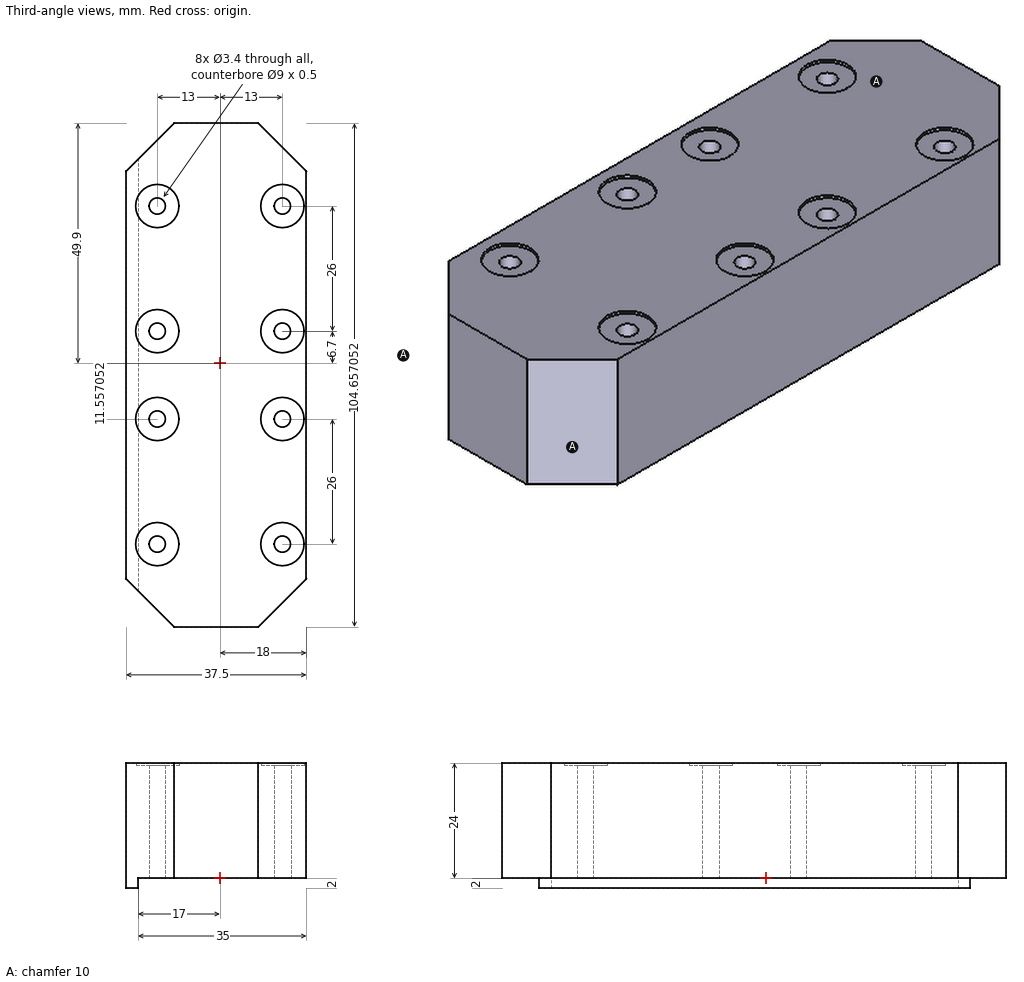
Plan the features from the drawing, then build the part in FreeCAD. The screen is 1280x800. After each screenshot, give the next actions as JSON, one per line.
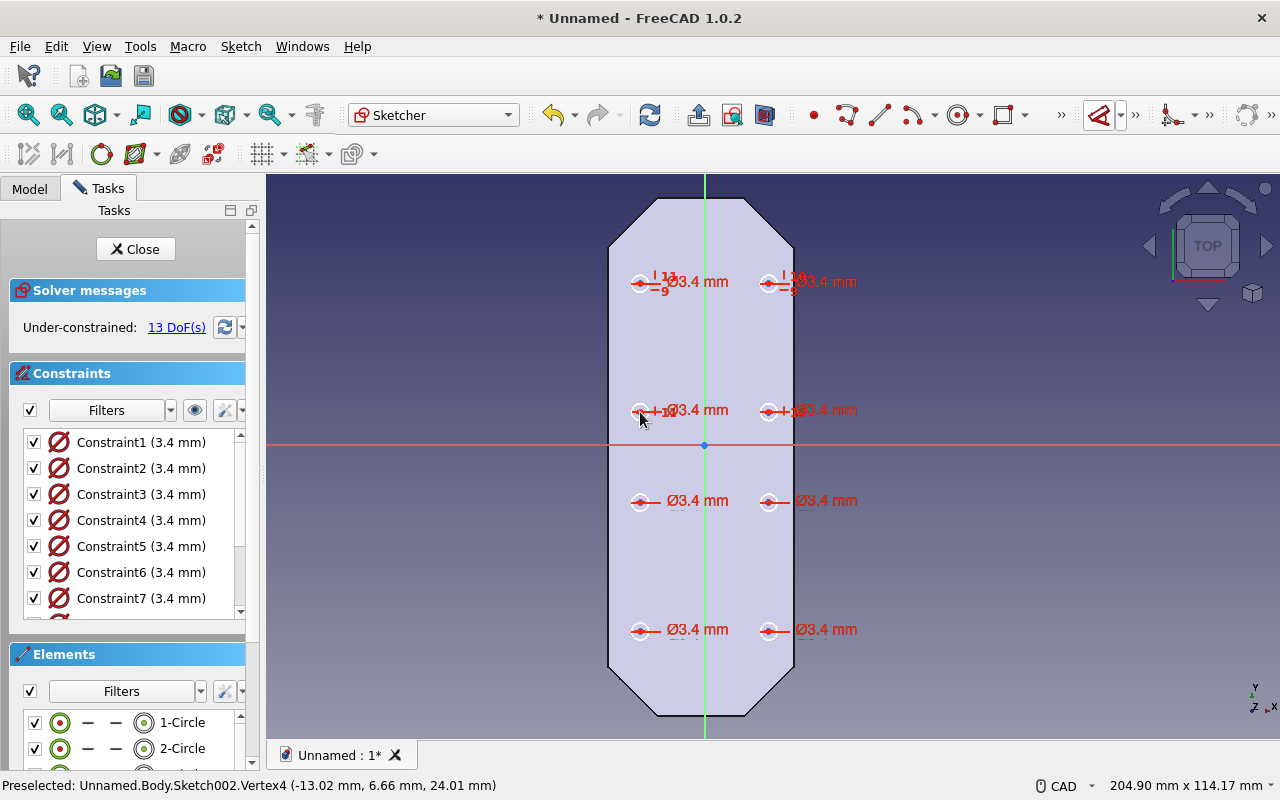
{"action": "left_click", "coordinate": [769, 412]}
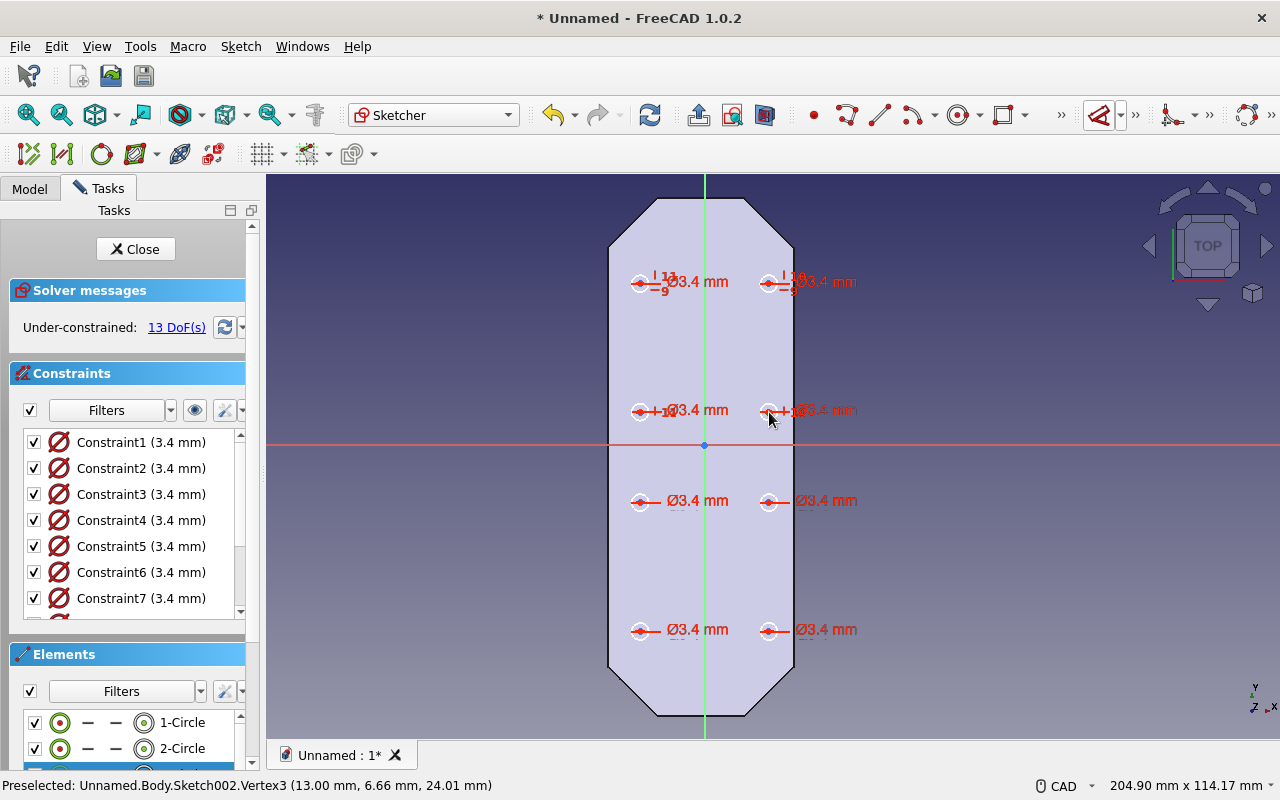
{"action": "left_click", "coordinate": [640, 412]}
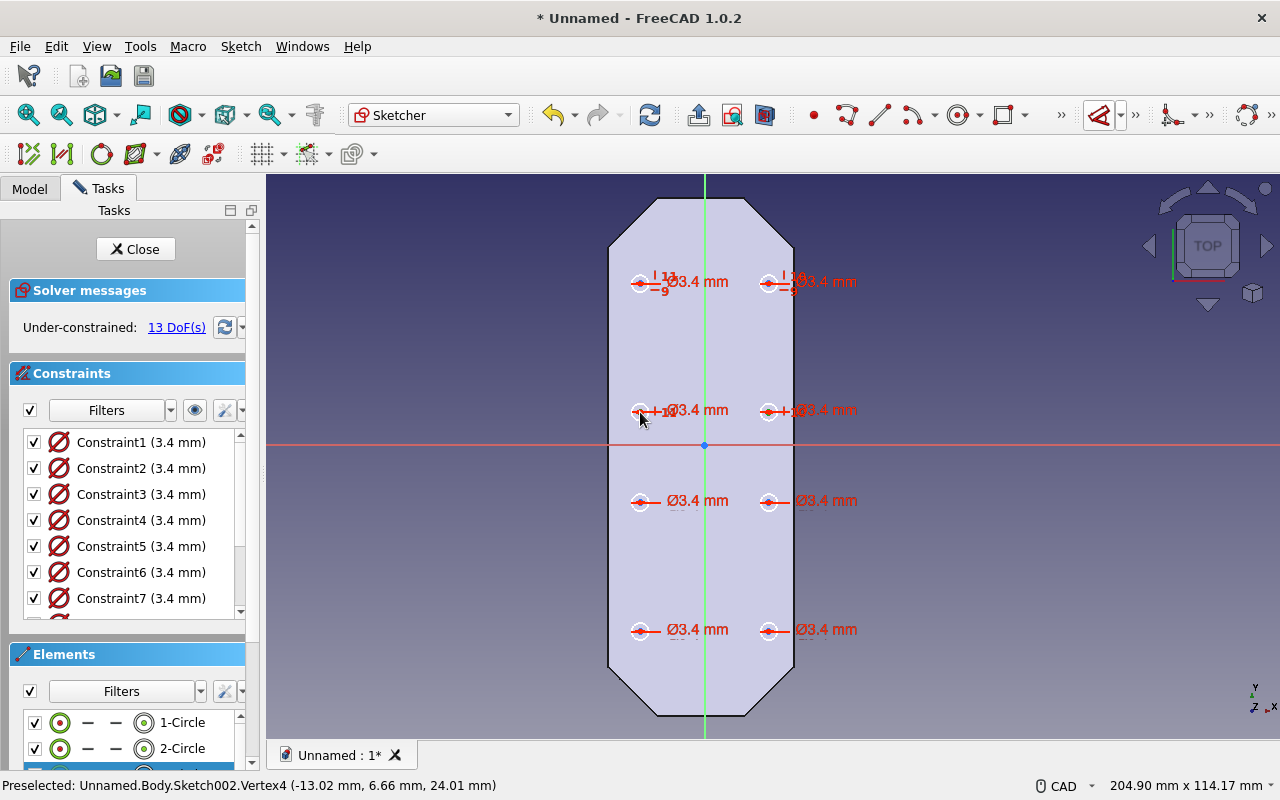
{"action": "key", "text": "h"}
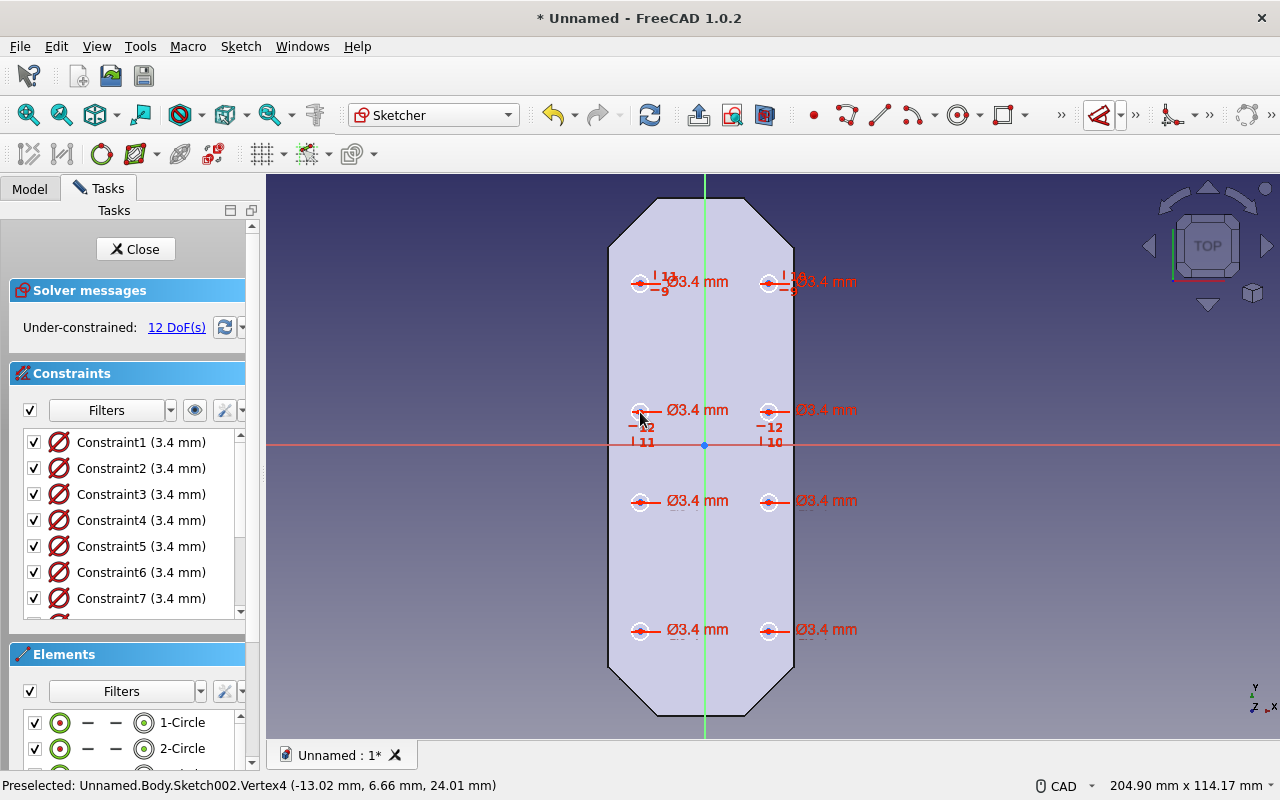
{"action": "left_click", "coordinate": [640, 412]}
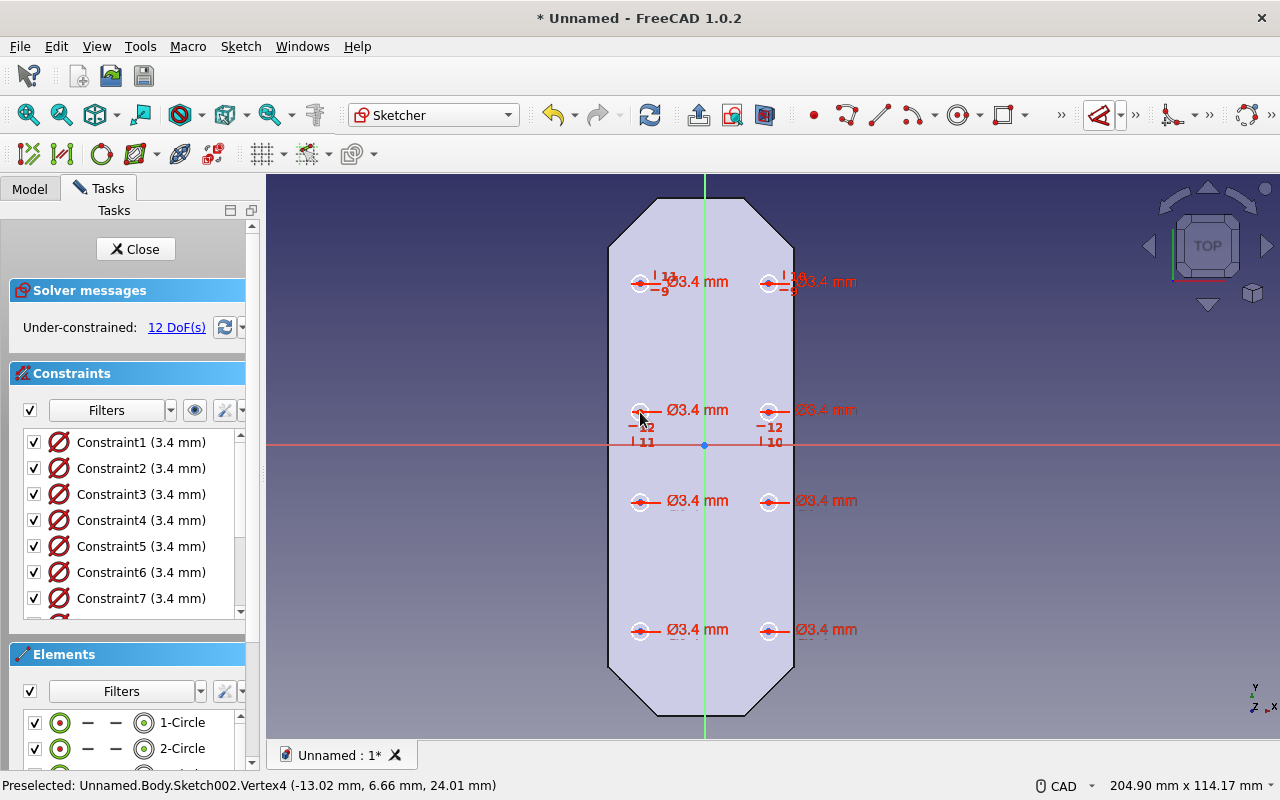
{"action": "left_click", "coordinate": [640, 503]}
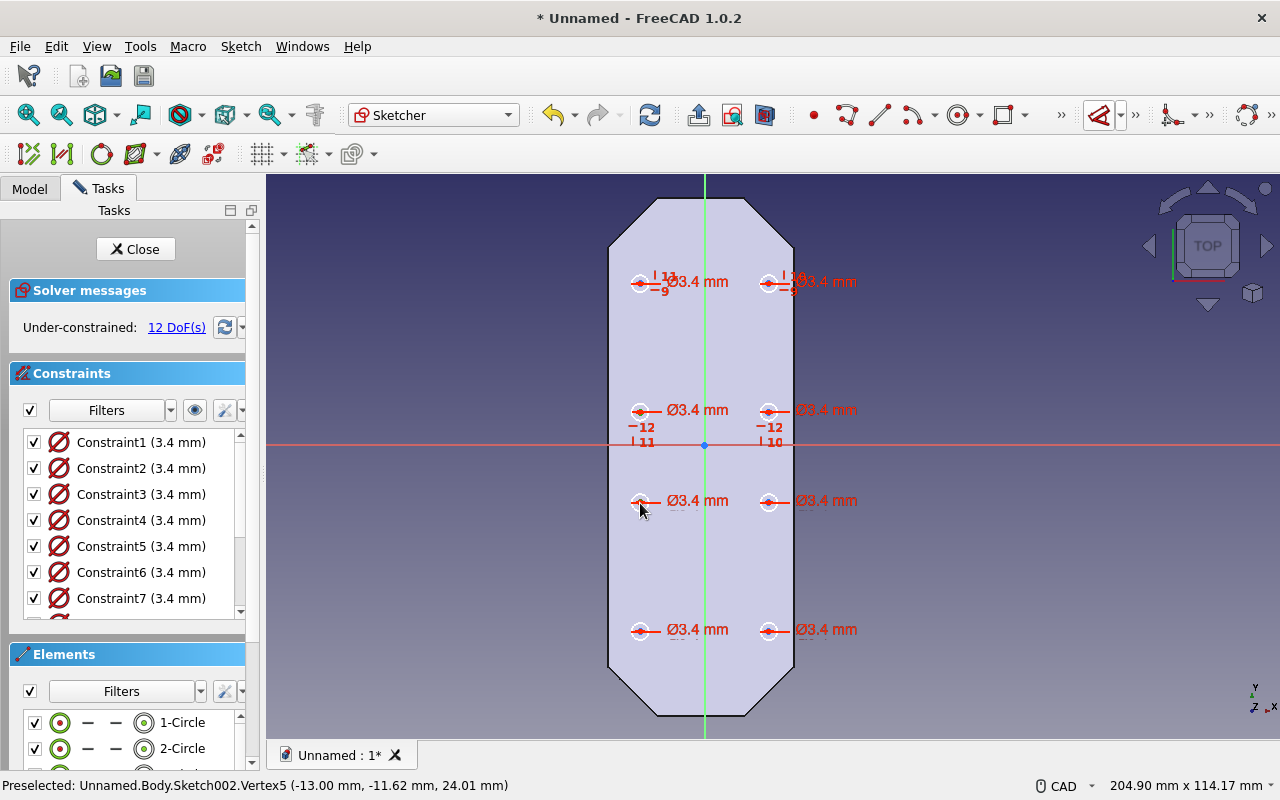
{"action": "key", "text": "v"}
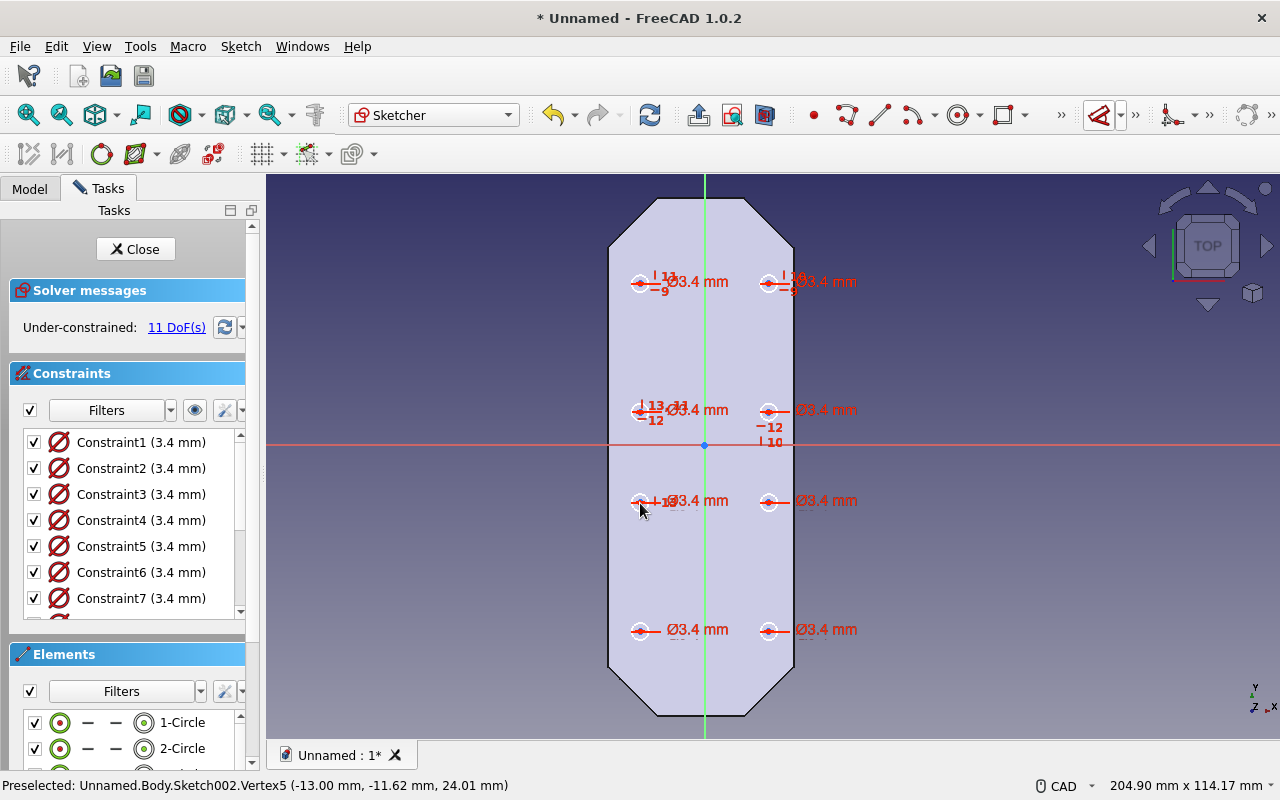
{"action": "left_click", "coordinate": [769, 412]}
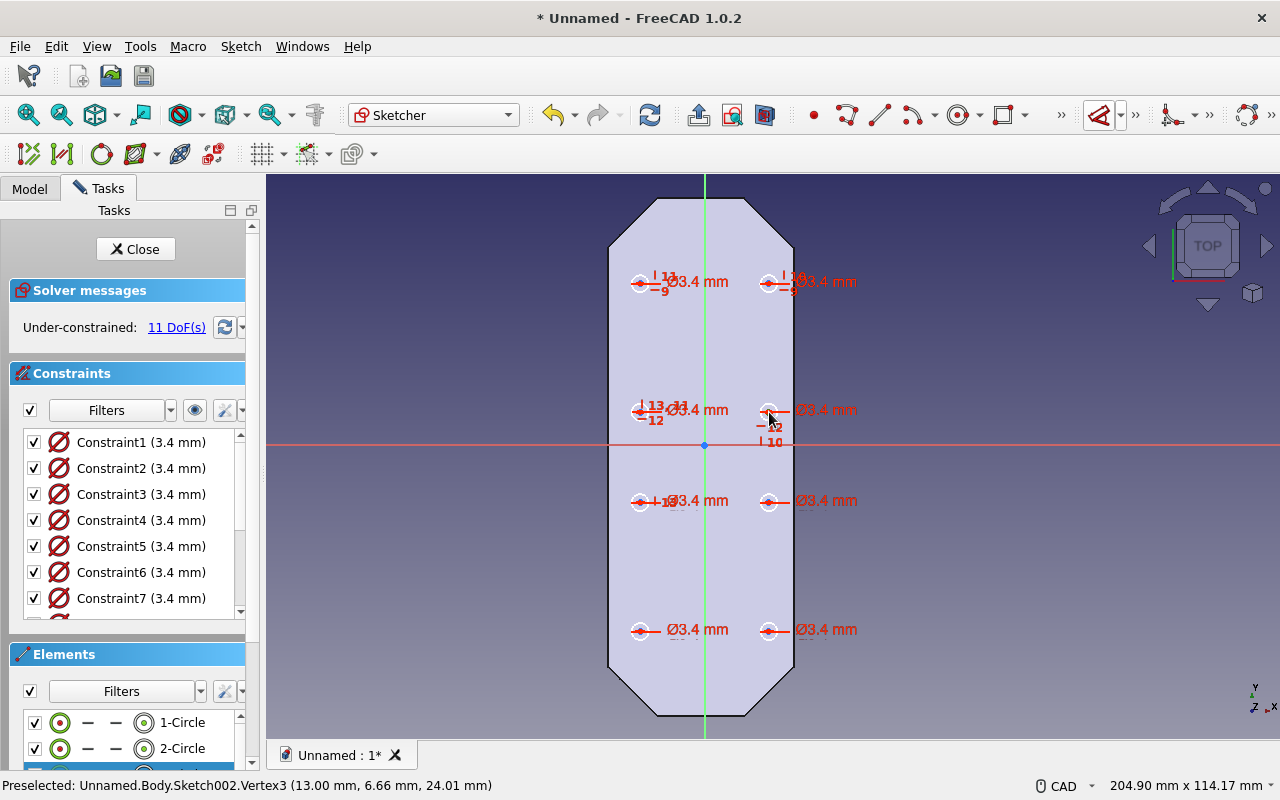
{"action": "left_click", "coordinate": [769, 503]}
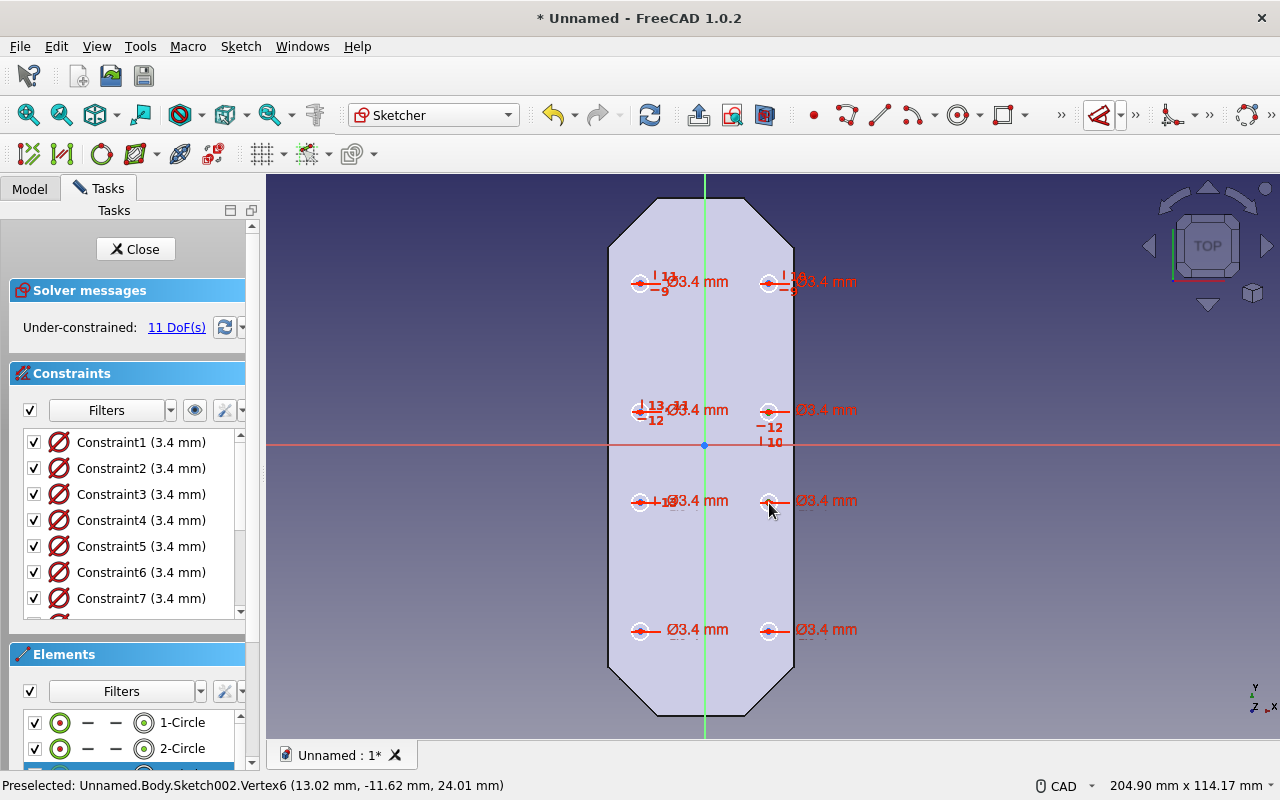
{"action": "key", "text": "v"}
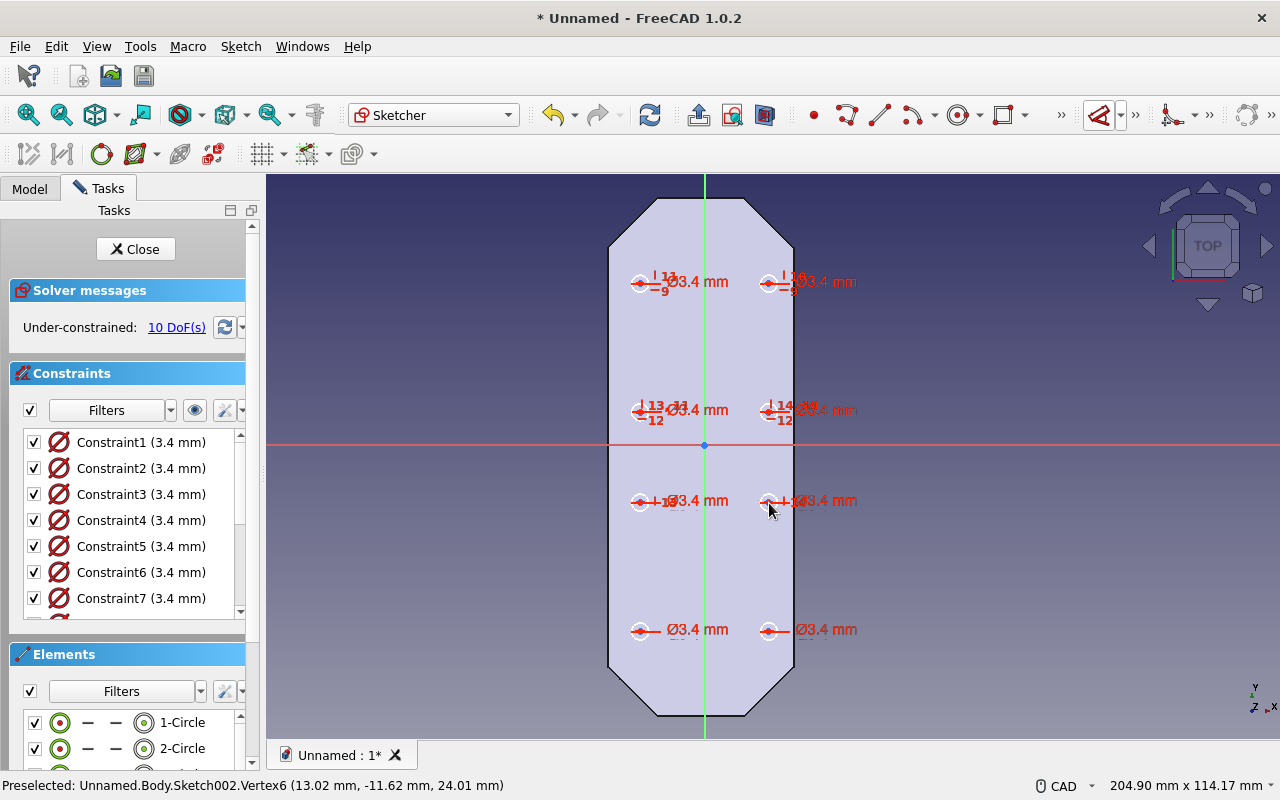
{"action": "left_click", "coordinate": [640, 503]}